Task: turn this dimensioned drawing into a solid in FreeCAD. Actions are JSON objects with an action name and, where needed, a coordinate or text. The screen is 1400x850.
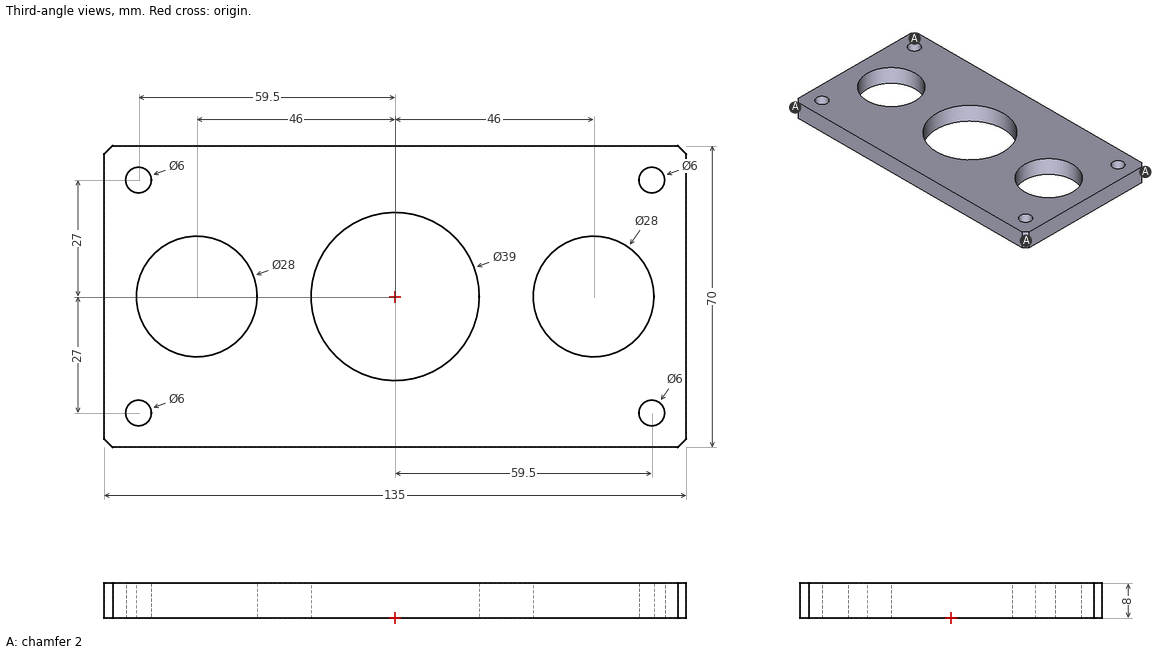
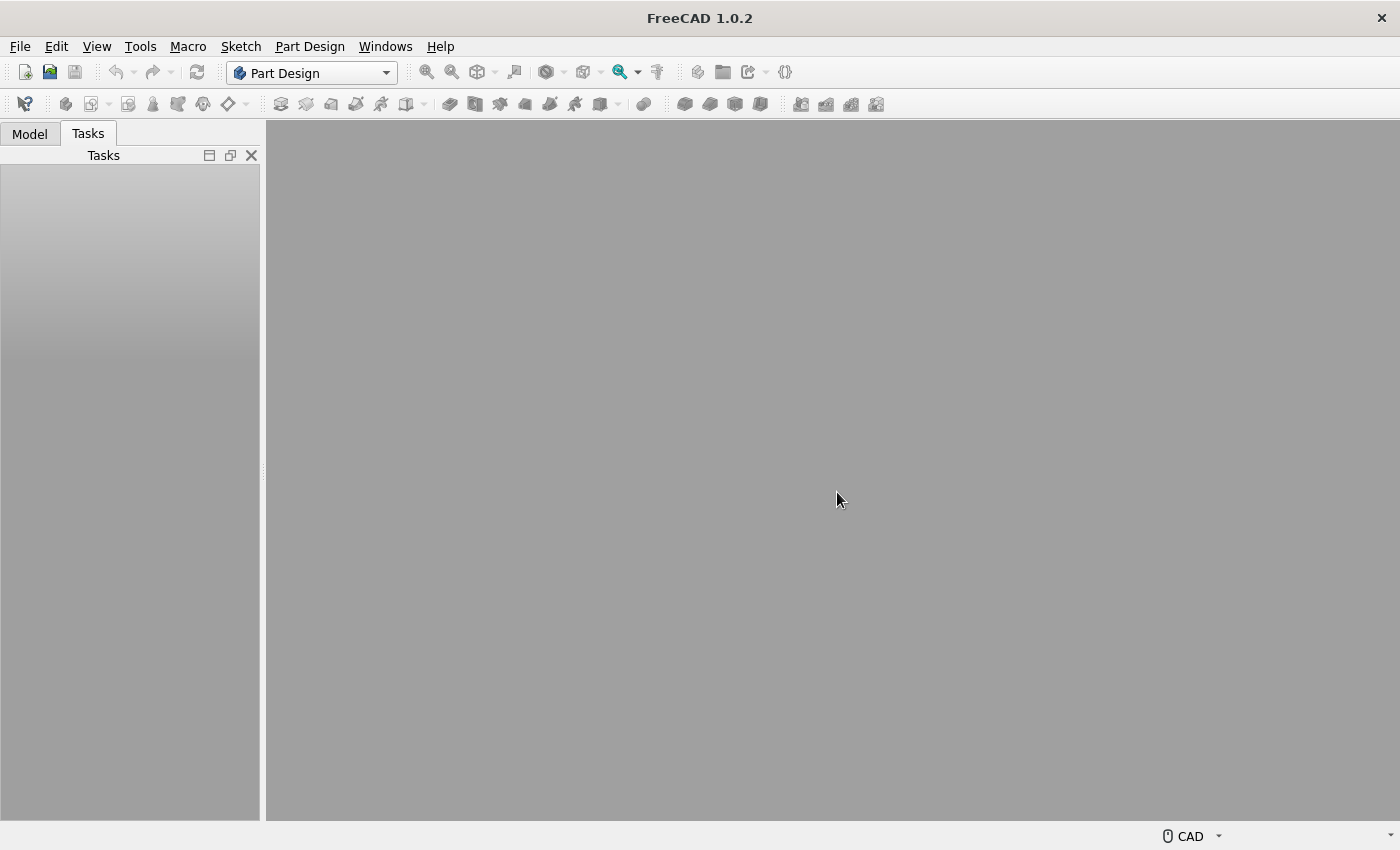
{"action": "key", "text": "ctrl+n"}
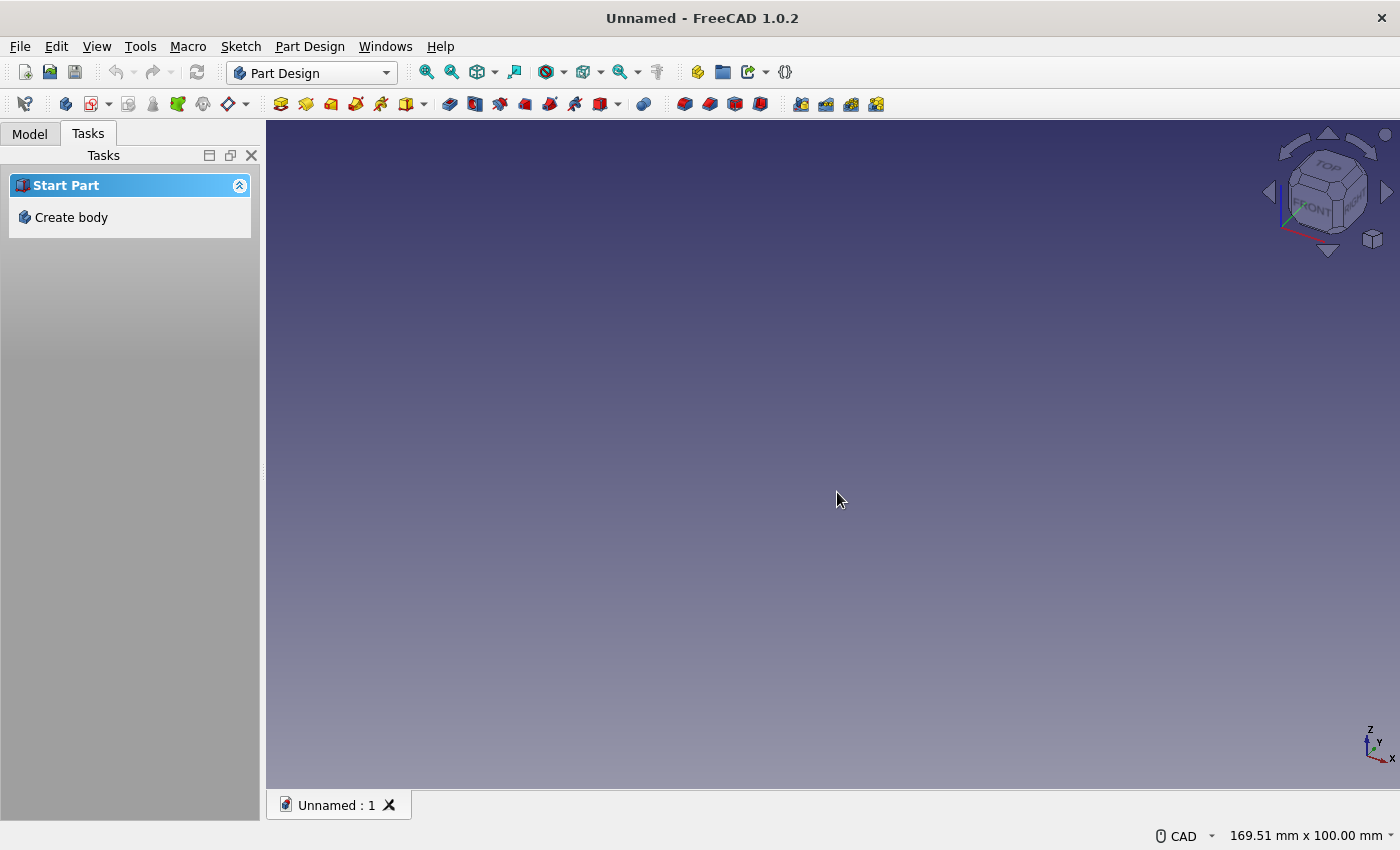
{"action": "left_click", "coordinate": [90, 104]}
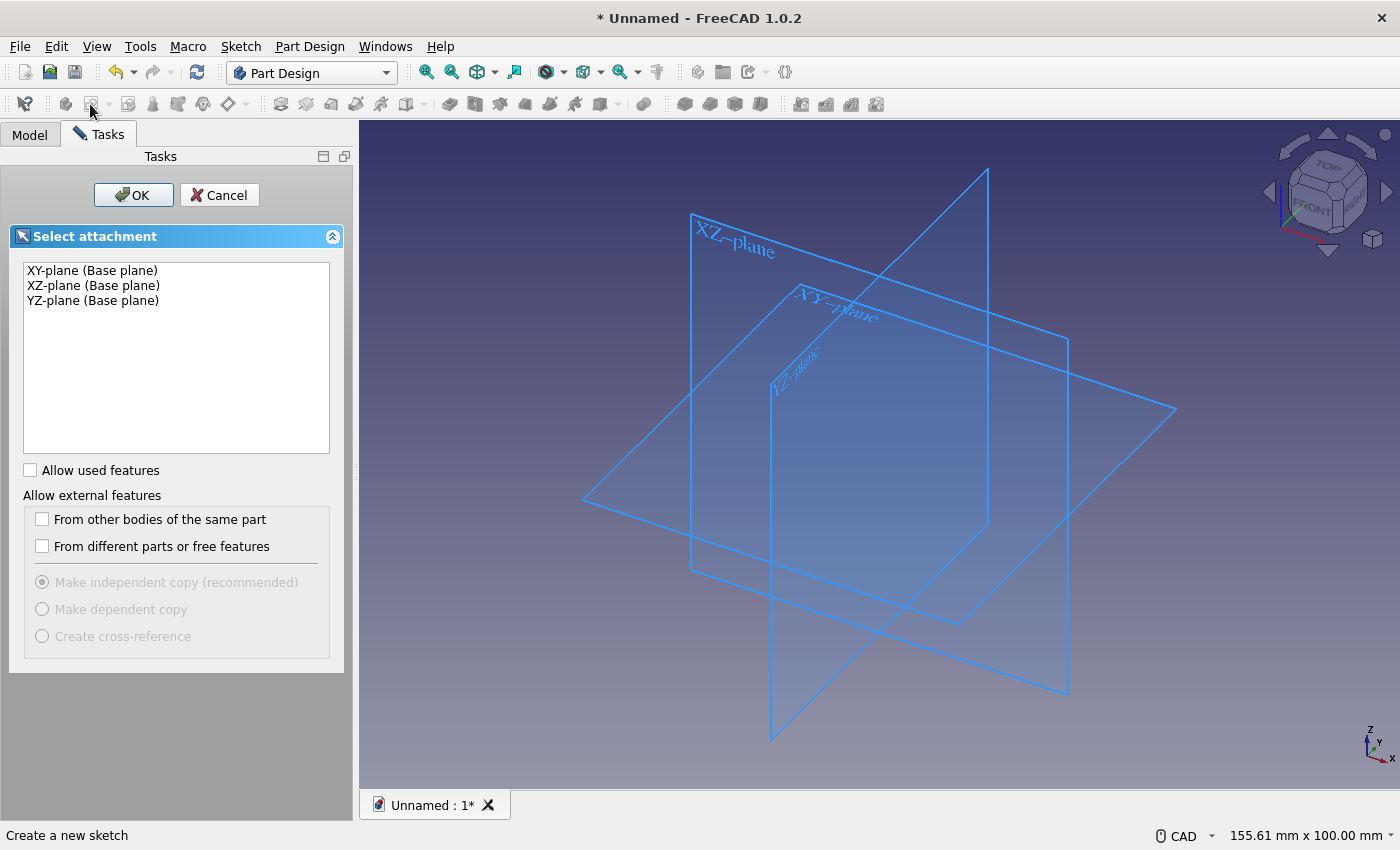
{"action": "left_click", "coordinate": [84, 270]}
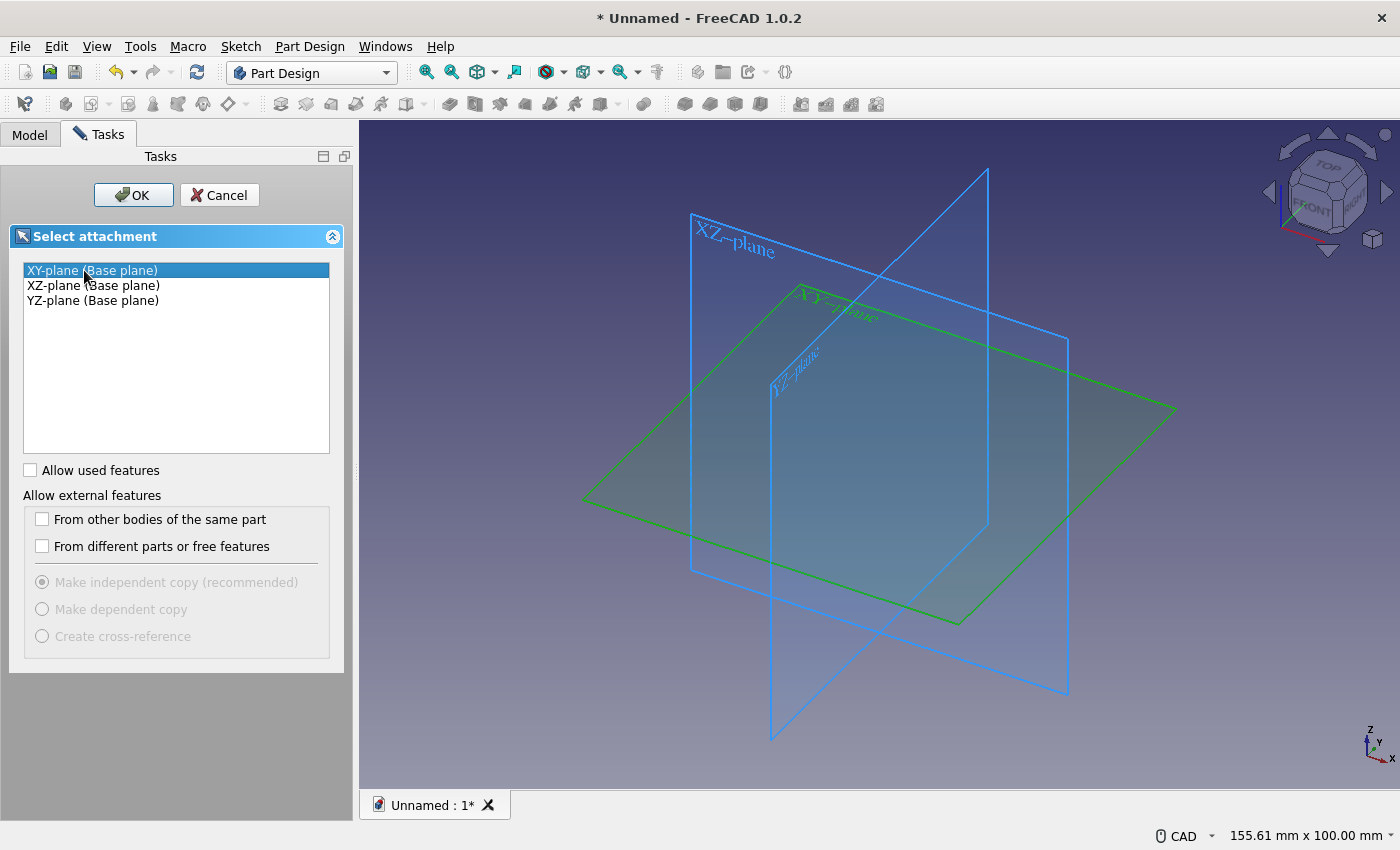
{"action": "left_click", "coordinate": [134, 195]}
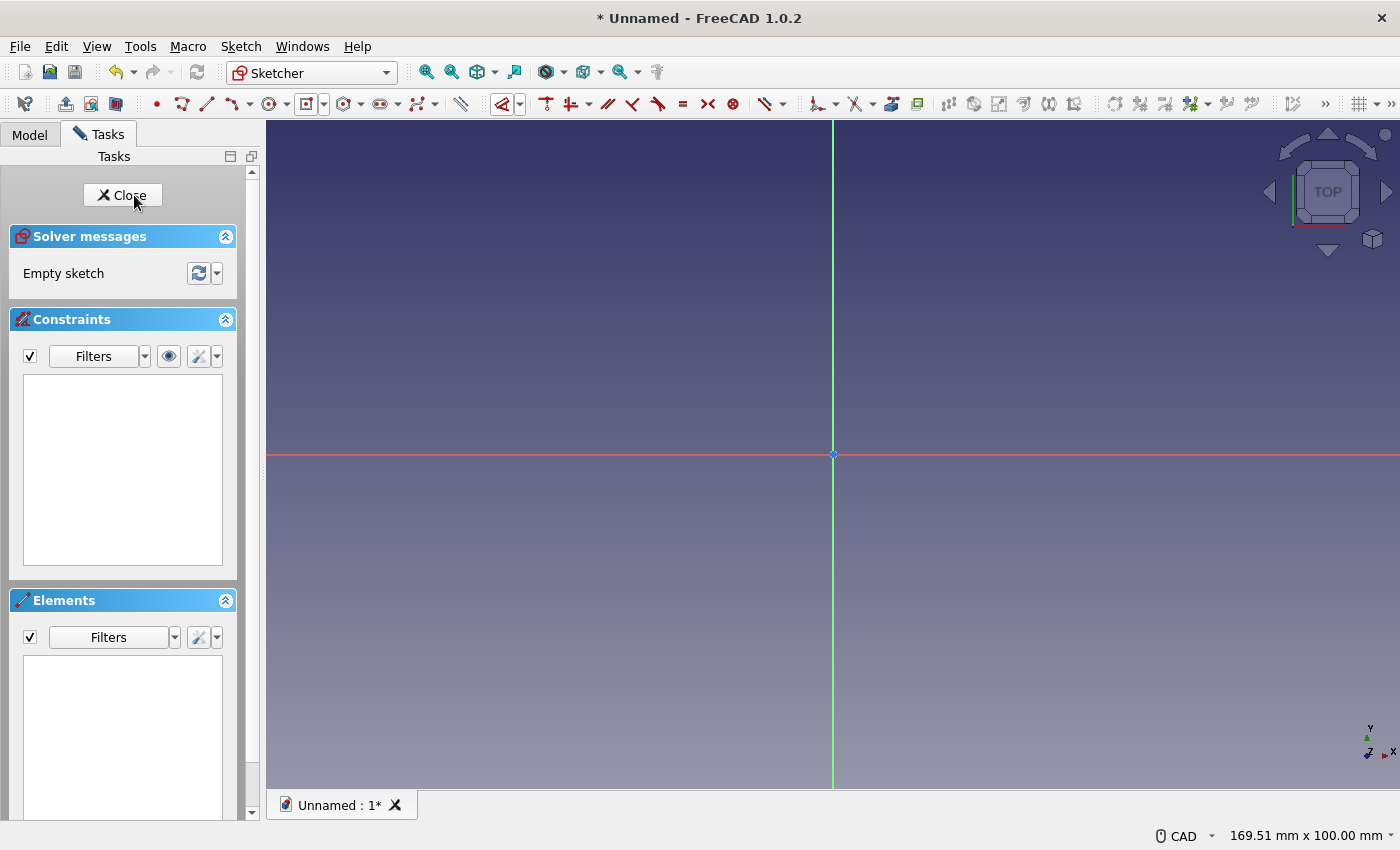
{"action": "scroll", "coordinate": [625, 455], "scroll_direction": "down", "scroll_amount": 2}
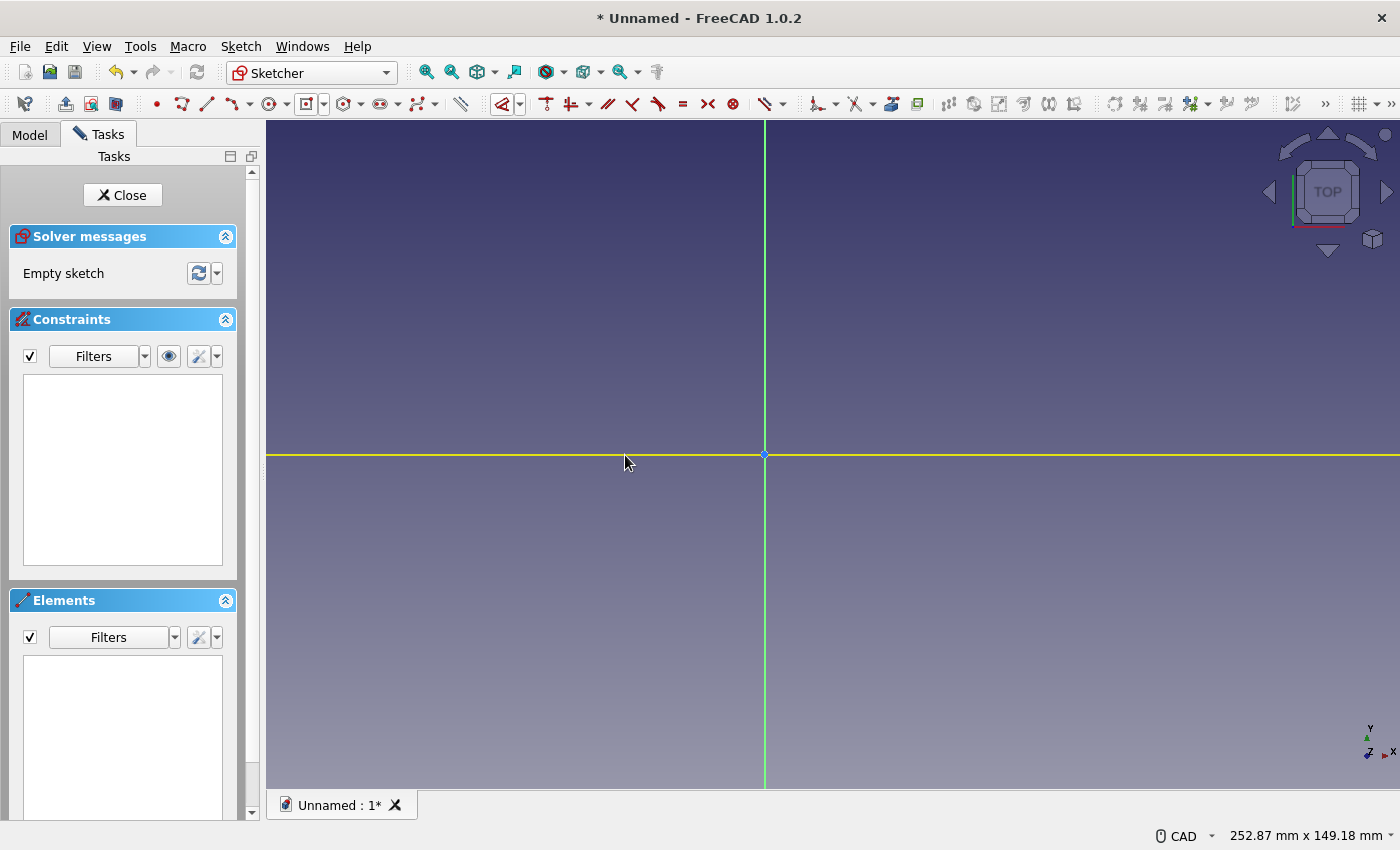
{"action": "left_click", "coordinate": [306, 104]}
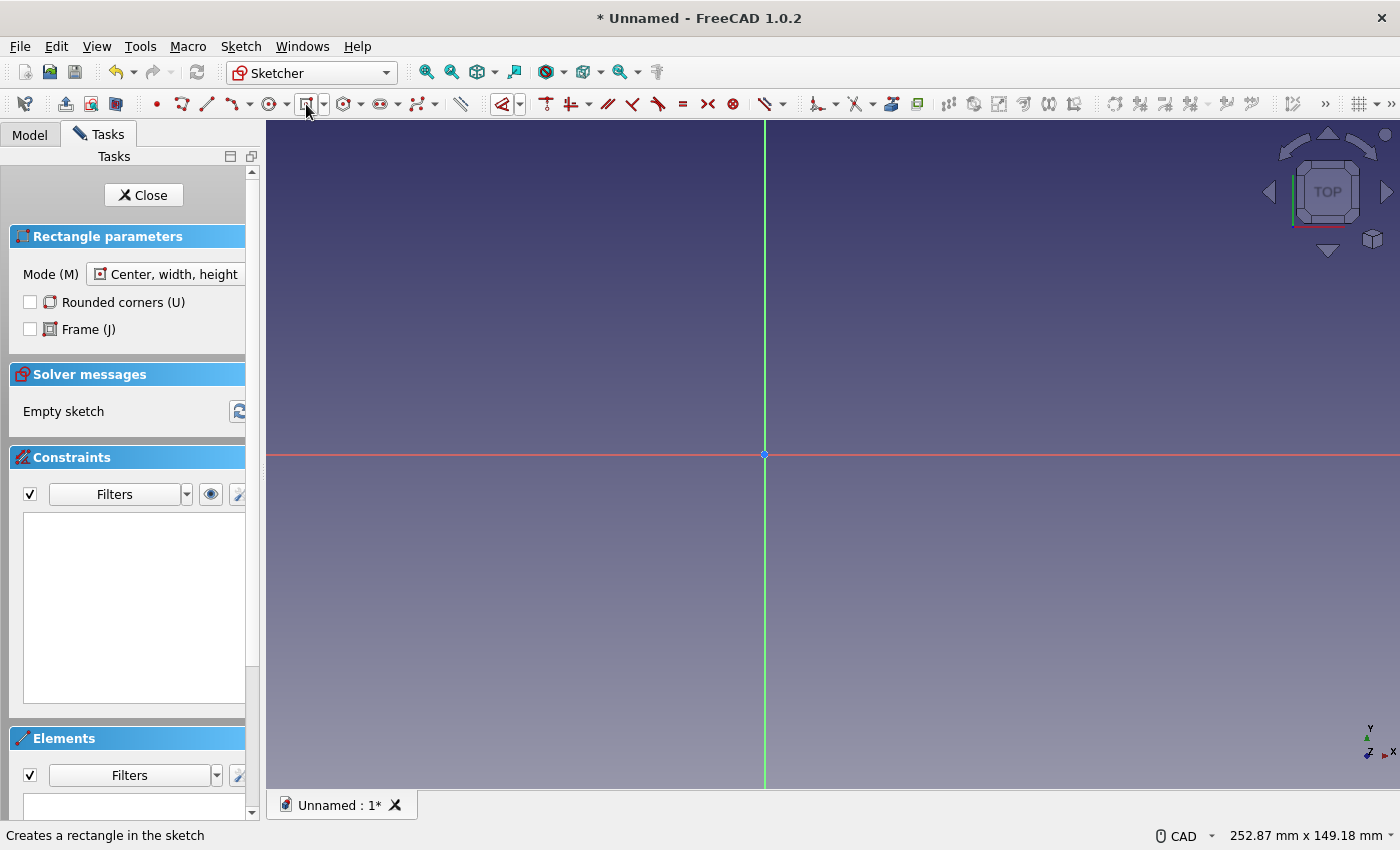
{"action": "left_click", "coordinate": [765, 455]}
{"action": "left_click", "coordinate": [1067, 298]}
{"action": "key", "text": "Escape"}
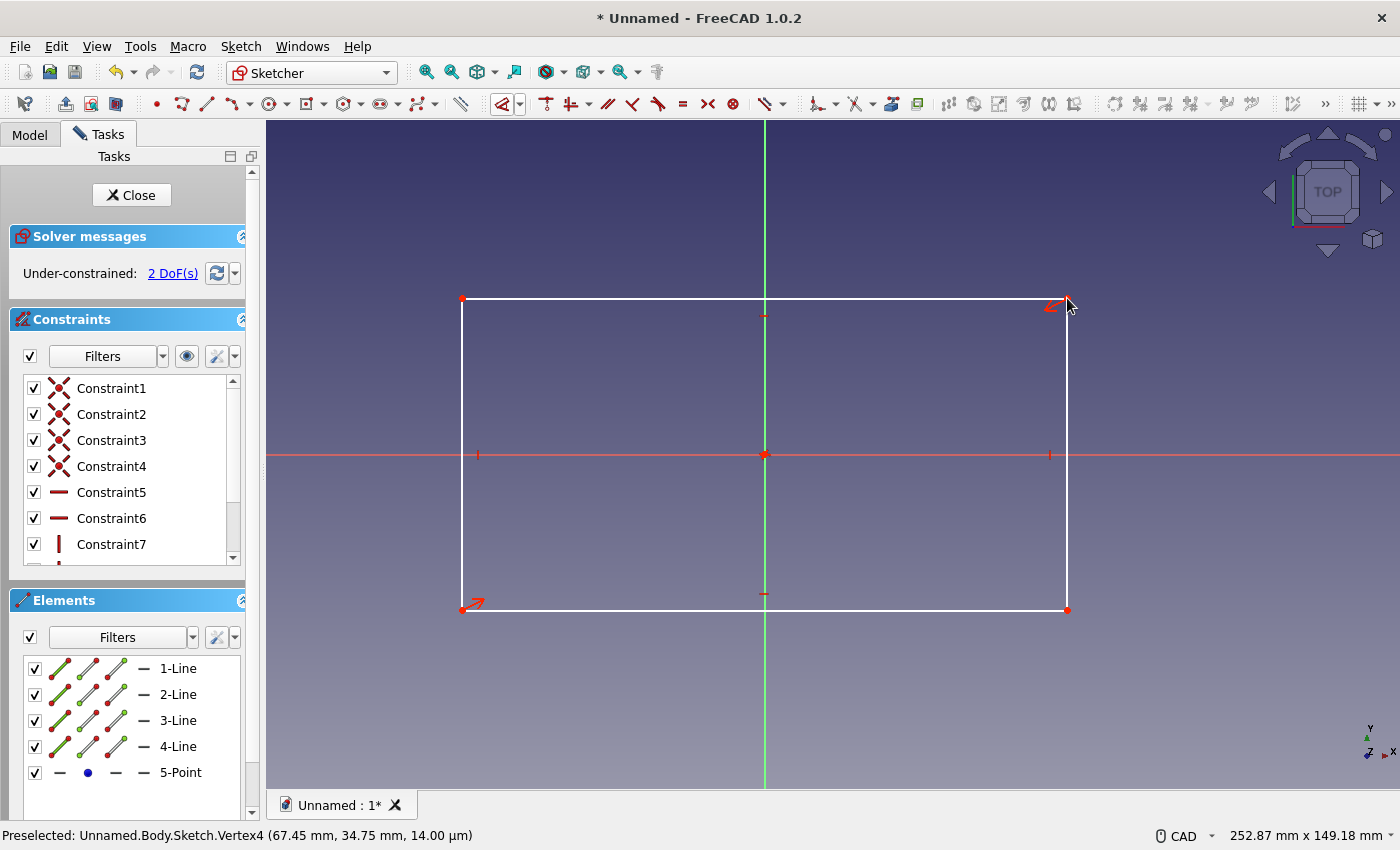
{"action": "left_click", "coordinate": [1067, 517]}